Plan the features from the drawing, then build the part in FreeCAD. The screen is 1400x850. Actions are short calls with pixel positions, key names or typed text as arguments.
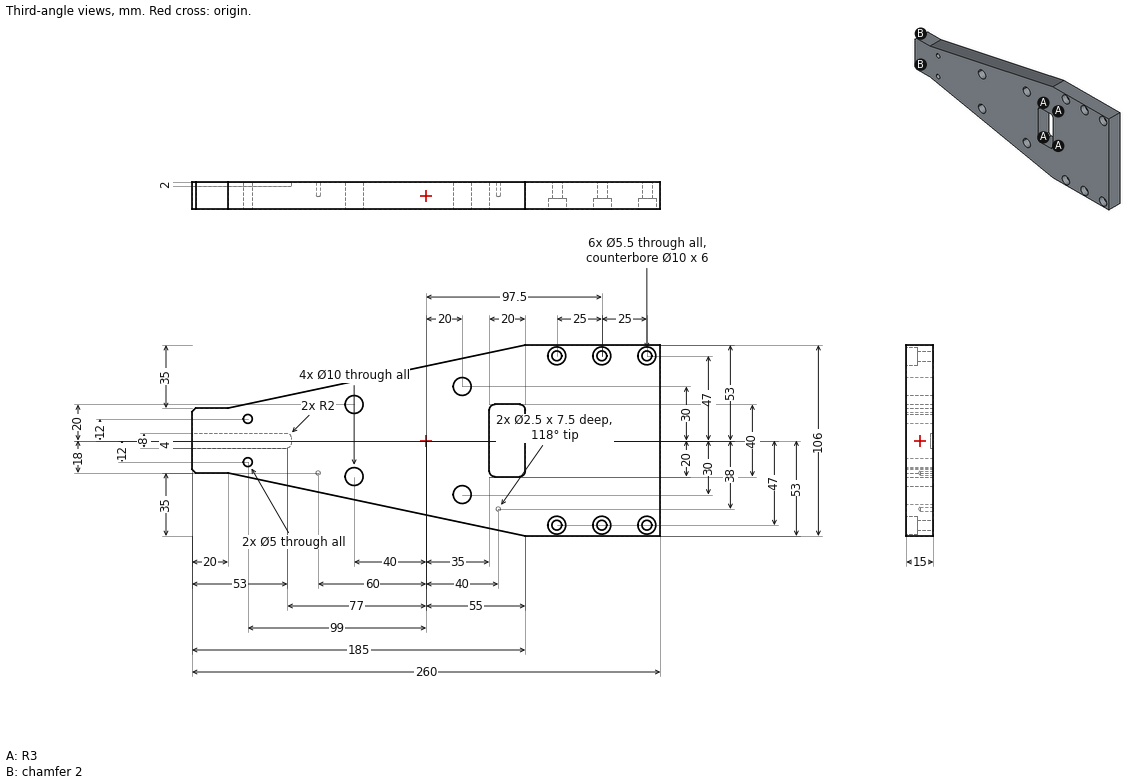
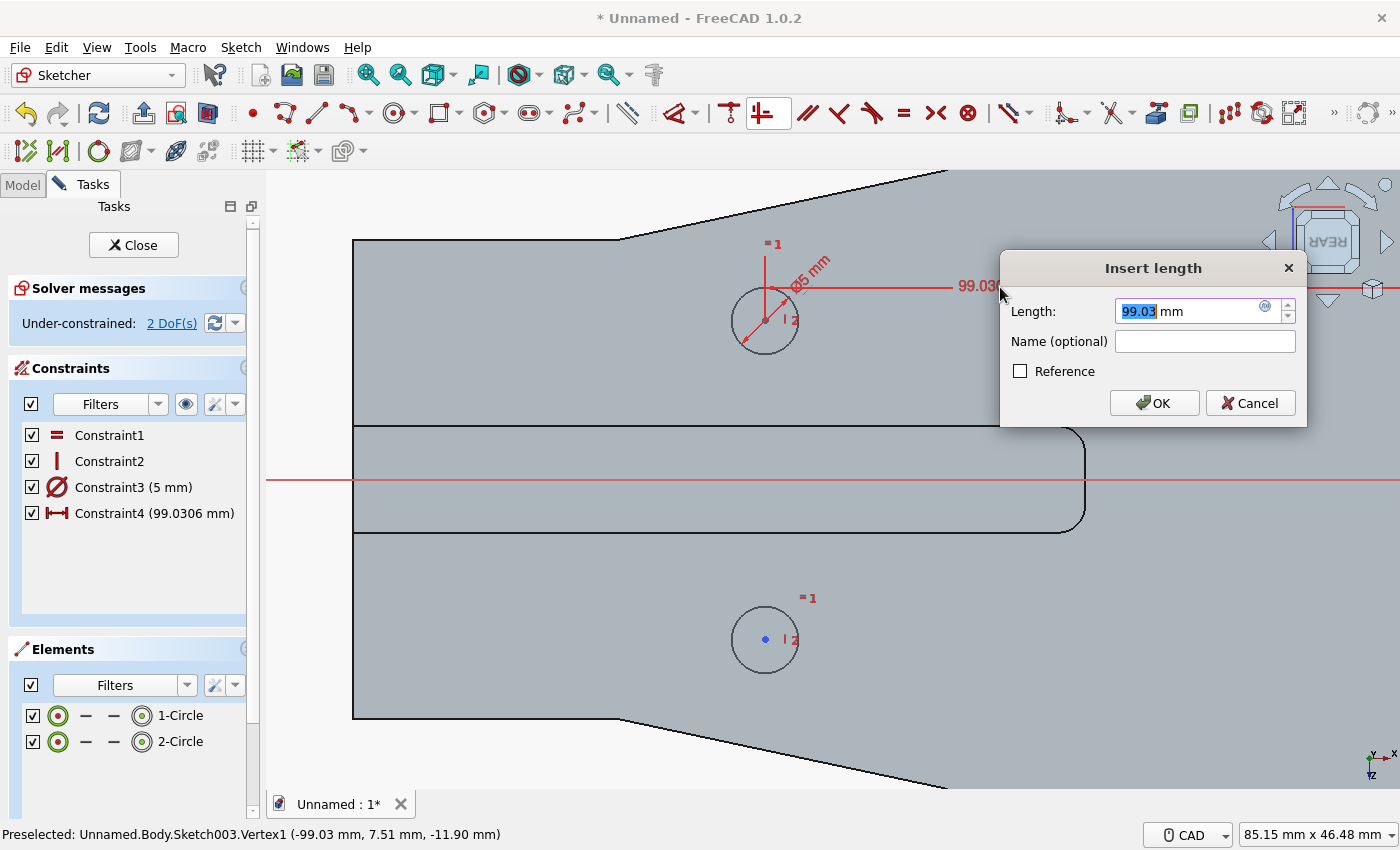
text(99)
key(Return)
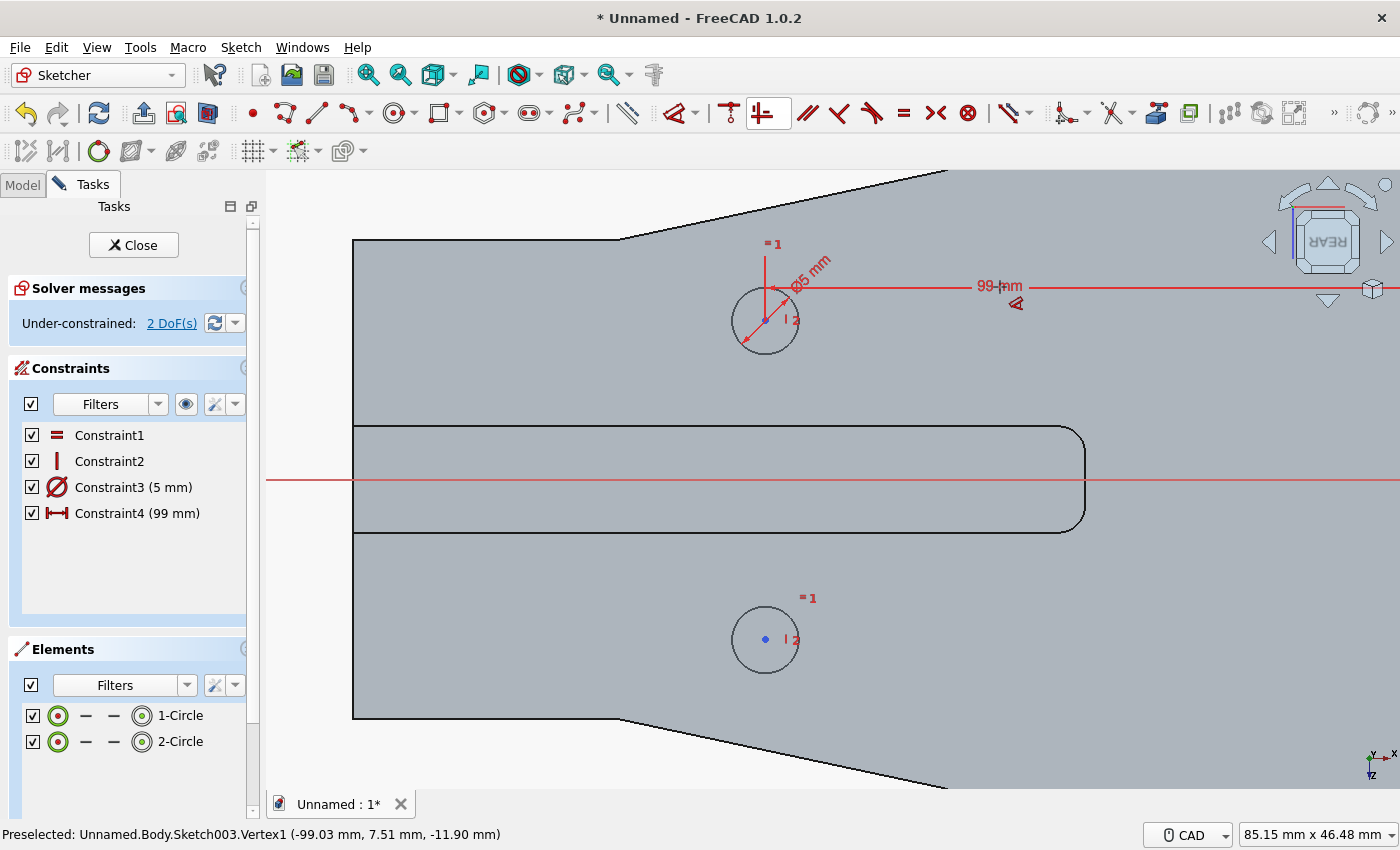
click(765, 321)
click(731, 400)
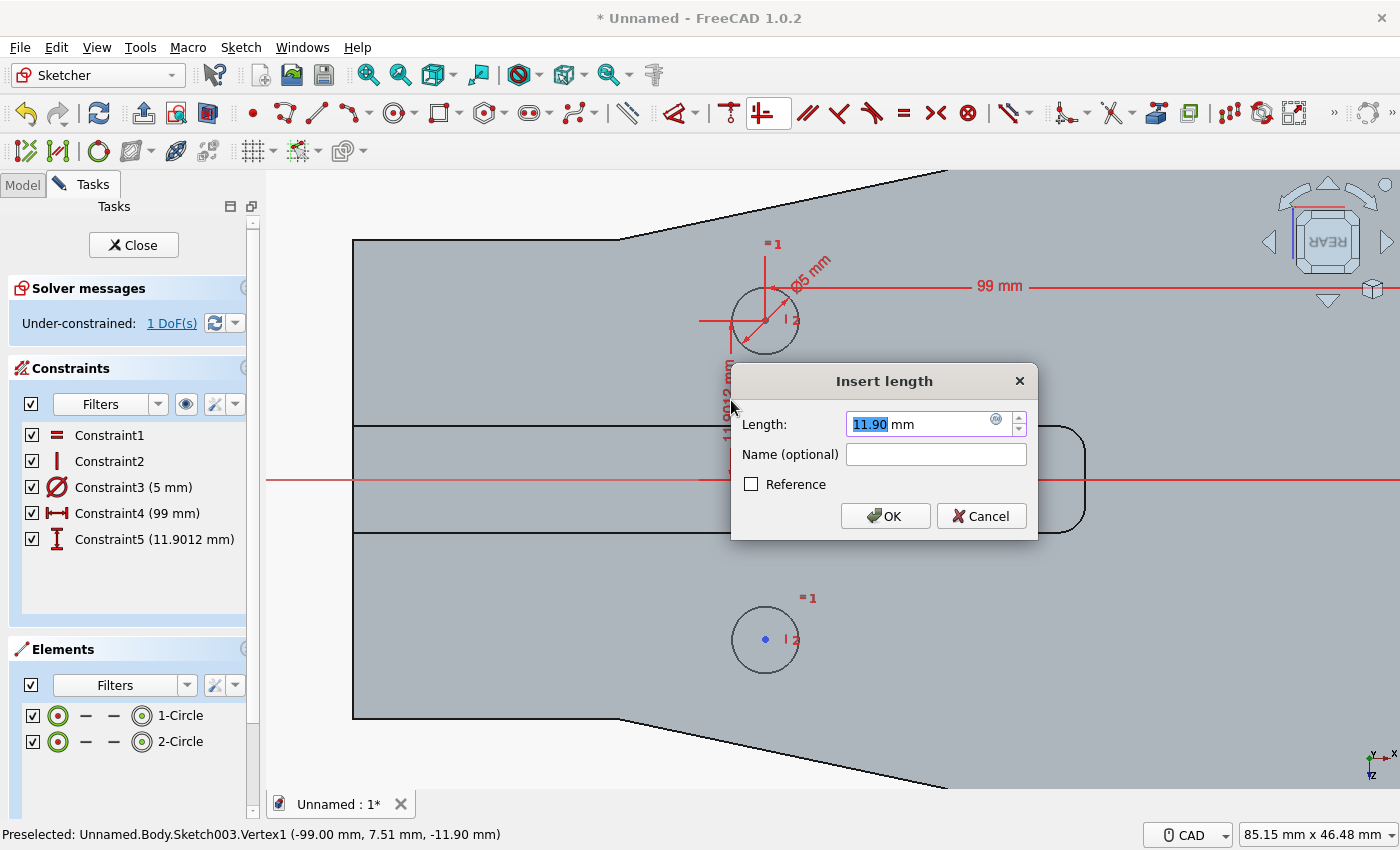
text(12)
key(Return)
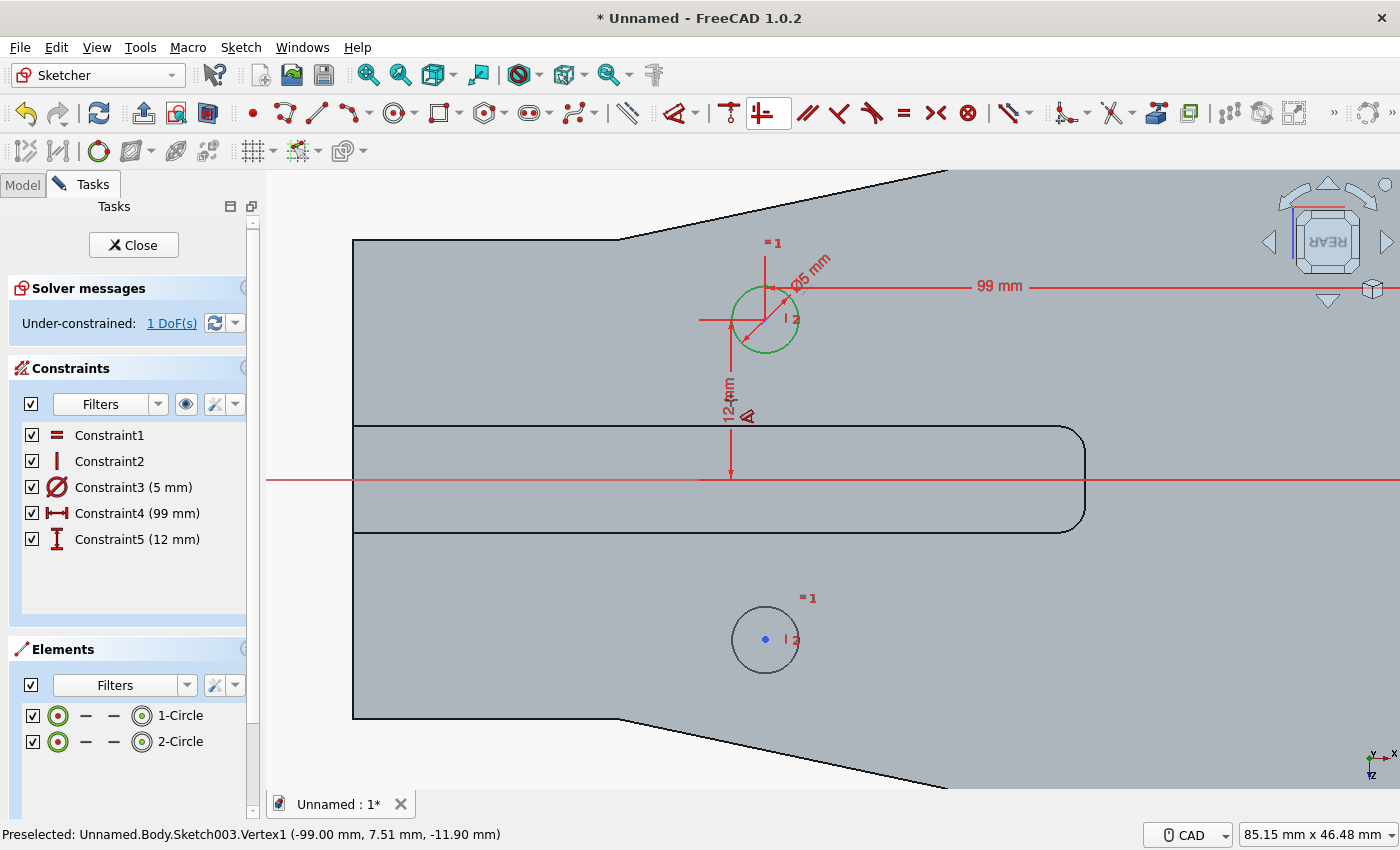
click(765, 640)
click(731, 560)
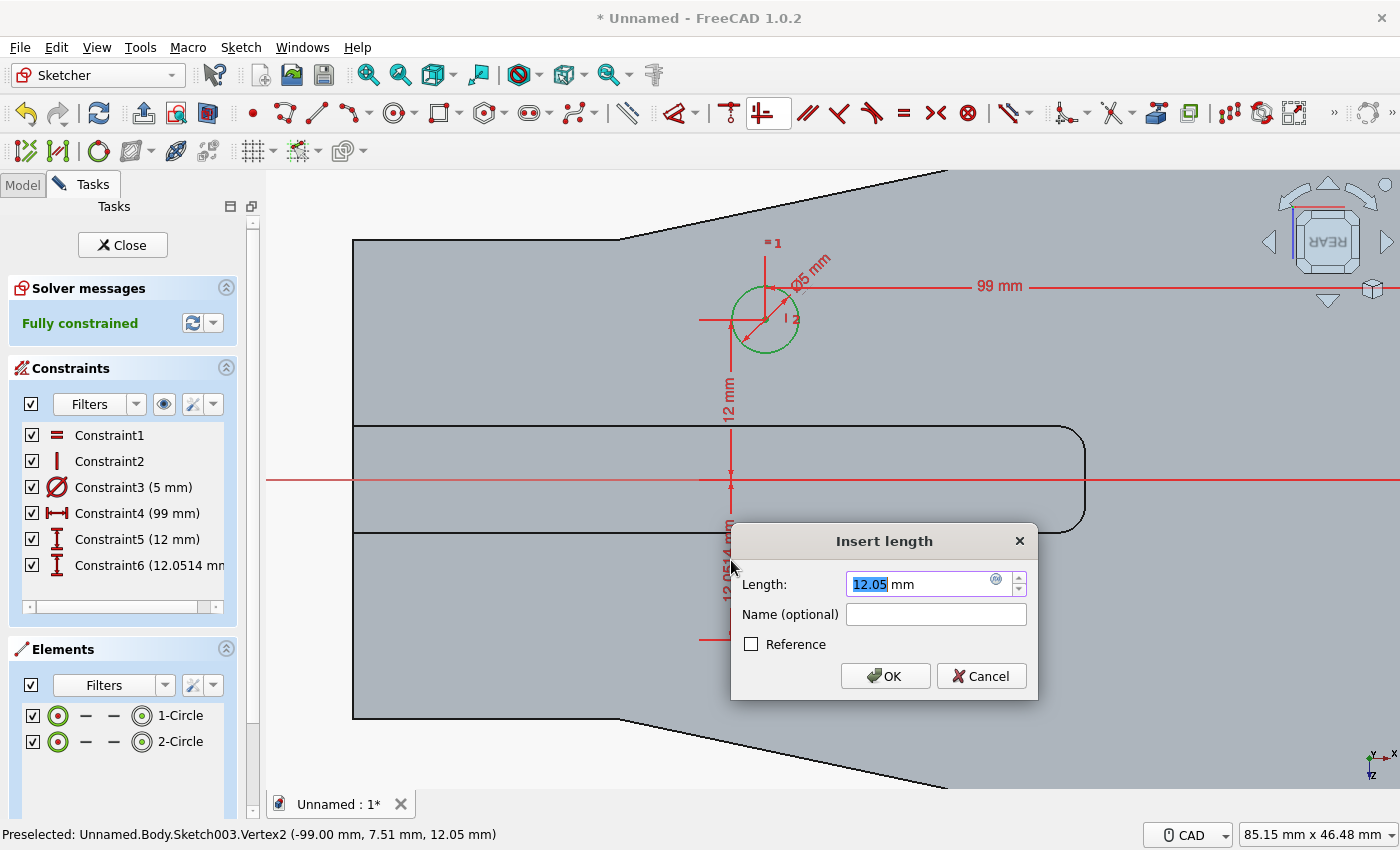
text(12)
key(Return)
key(Escape)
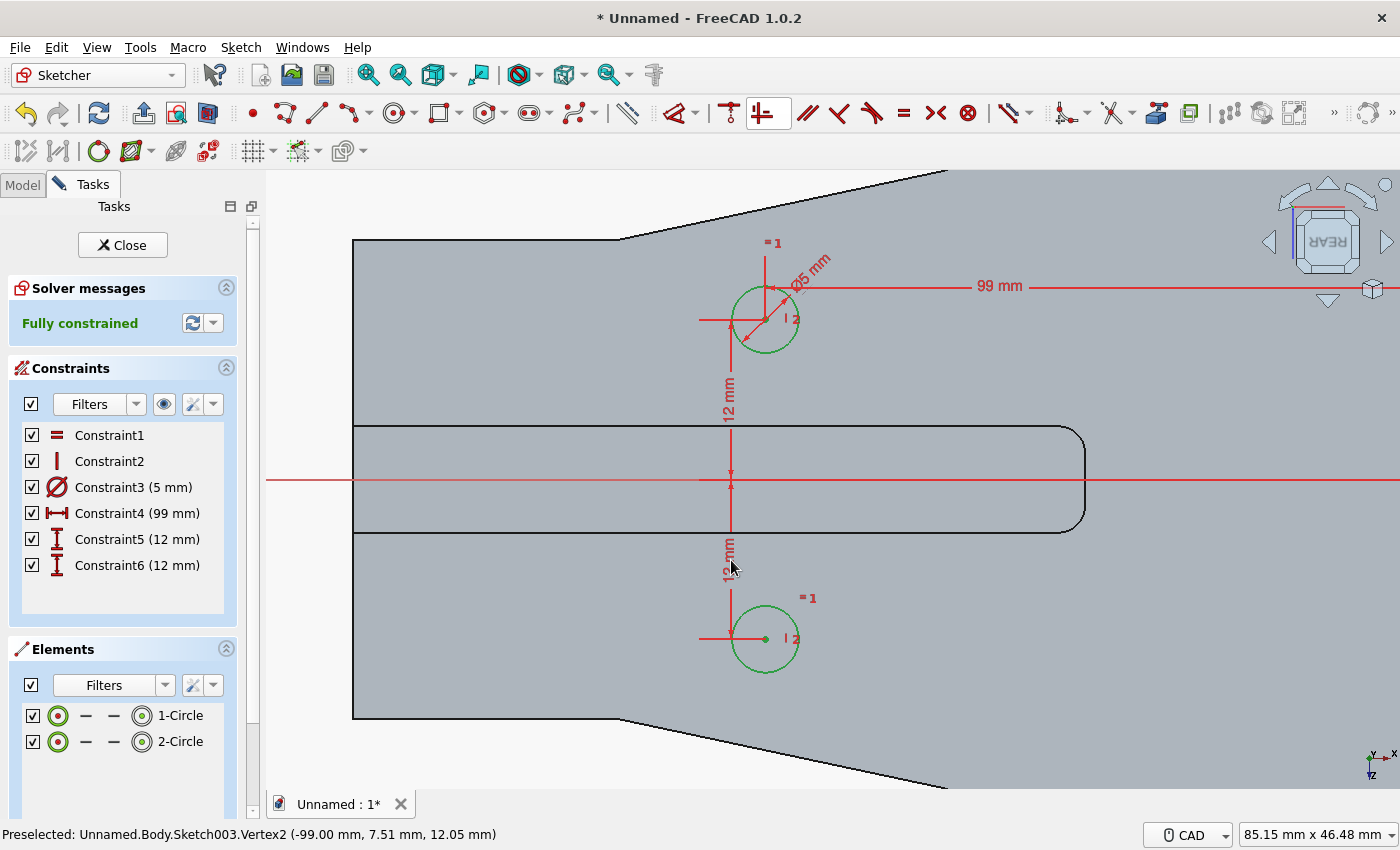
click(123, 245)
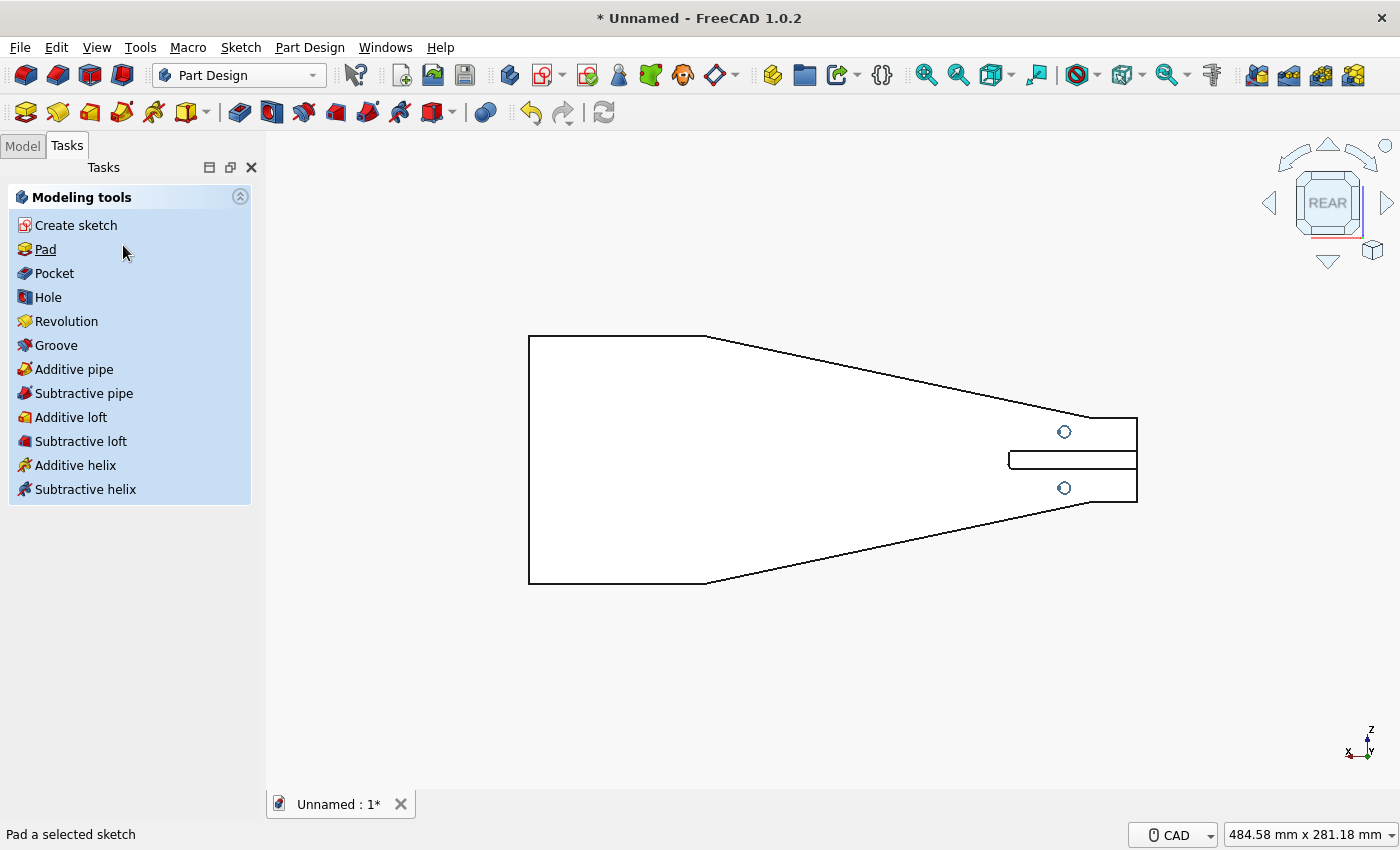
click(272, 112)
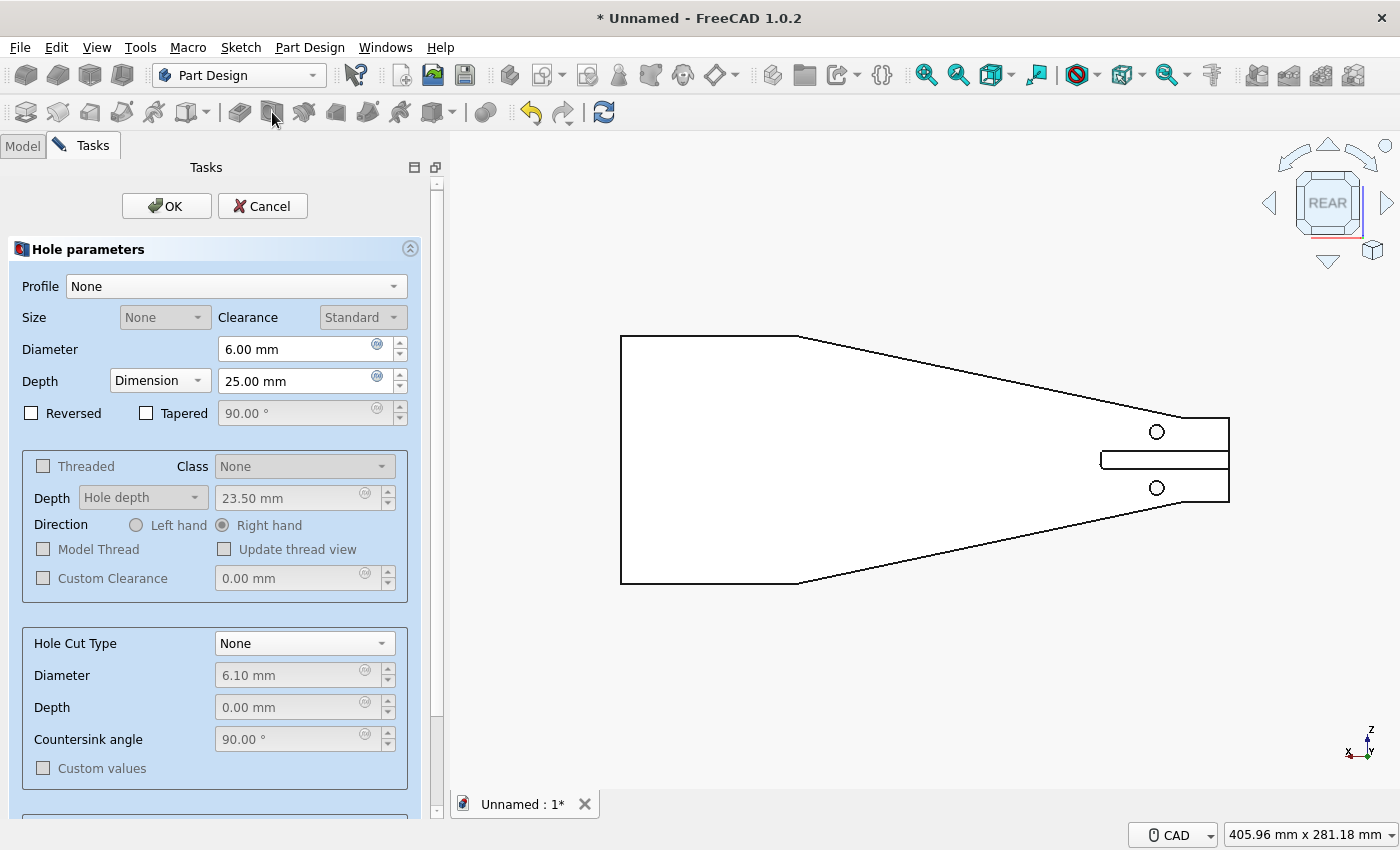
triple_click(305, 349)